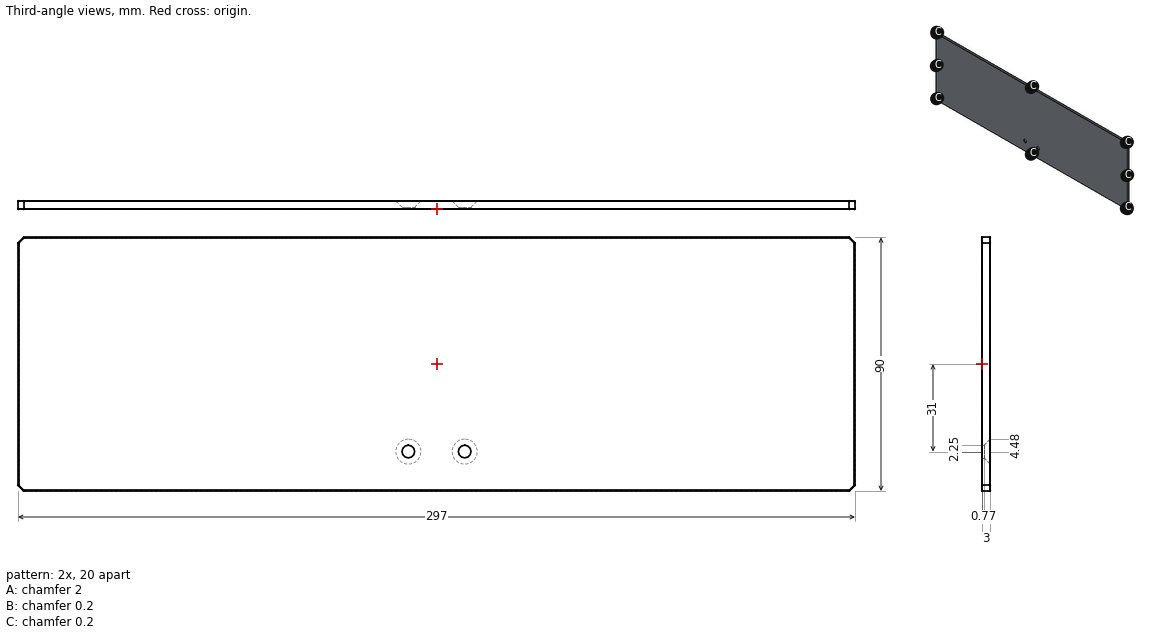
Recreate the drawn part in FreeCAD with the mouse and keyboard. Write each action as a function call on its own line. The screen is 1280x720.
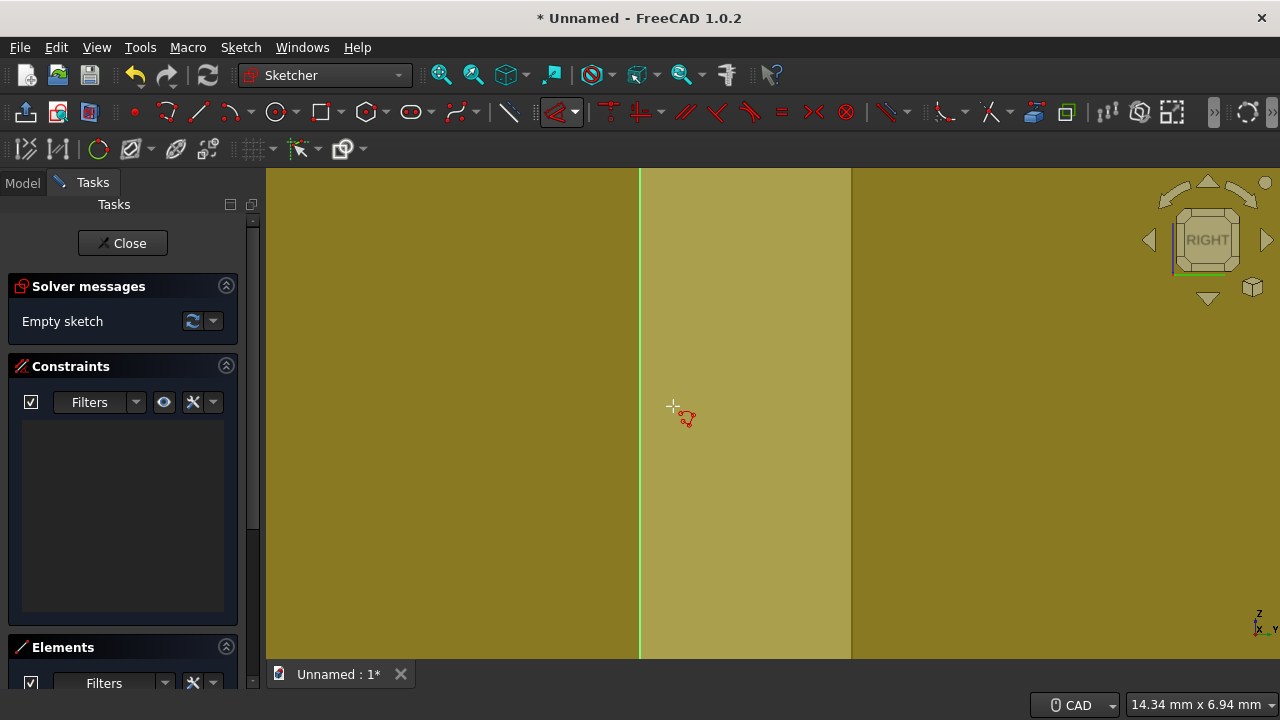
click(852, 255)
click(695, 412)
click(640, 412)
click(649, 571)
click(852, 571)
click(852, 256)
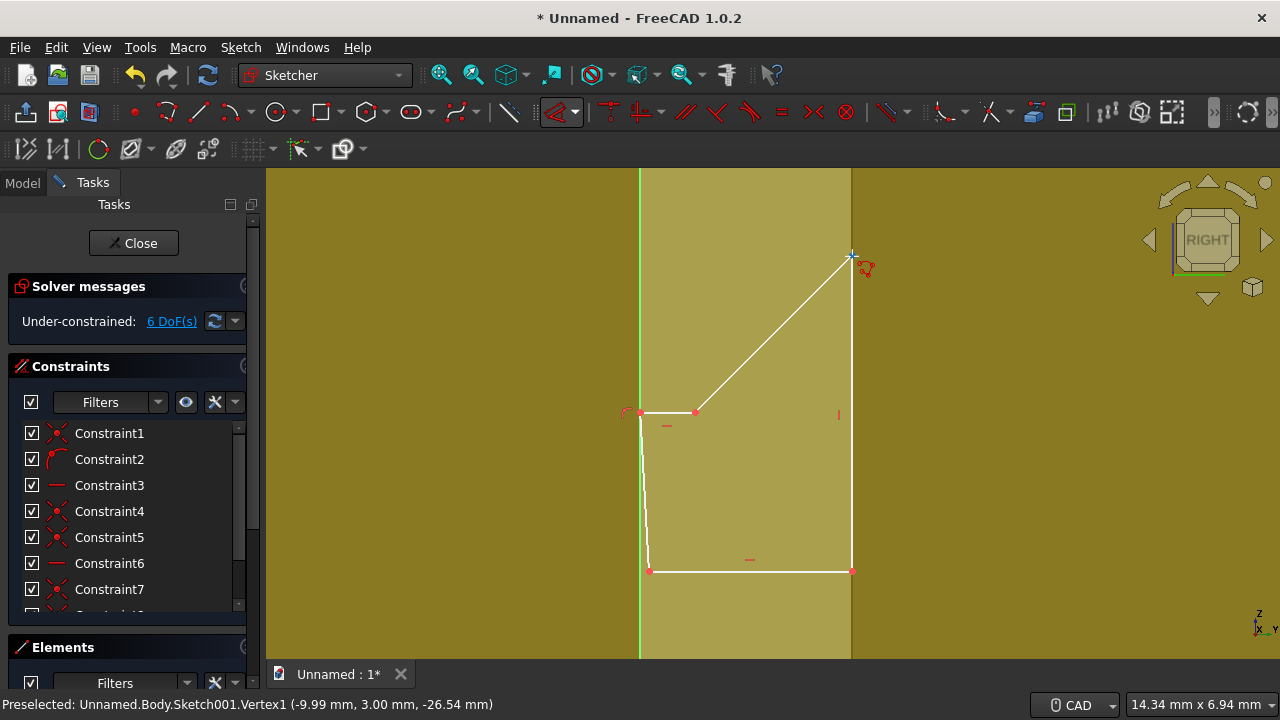
key(g)
key(l)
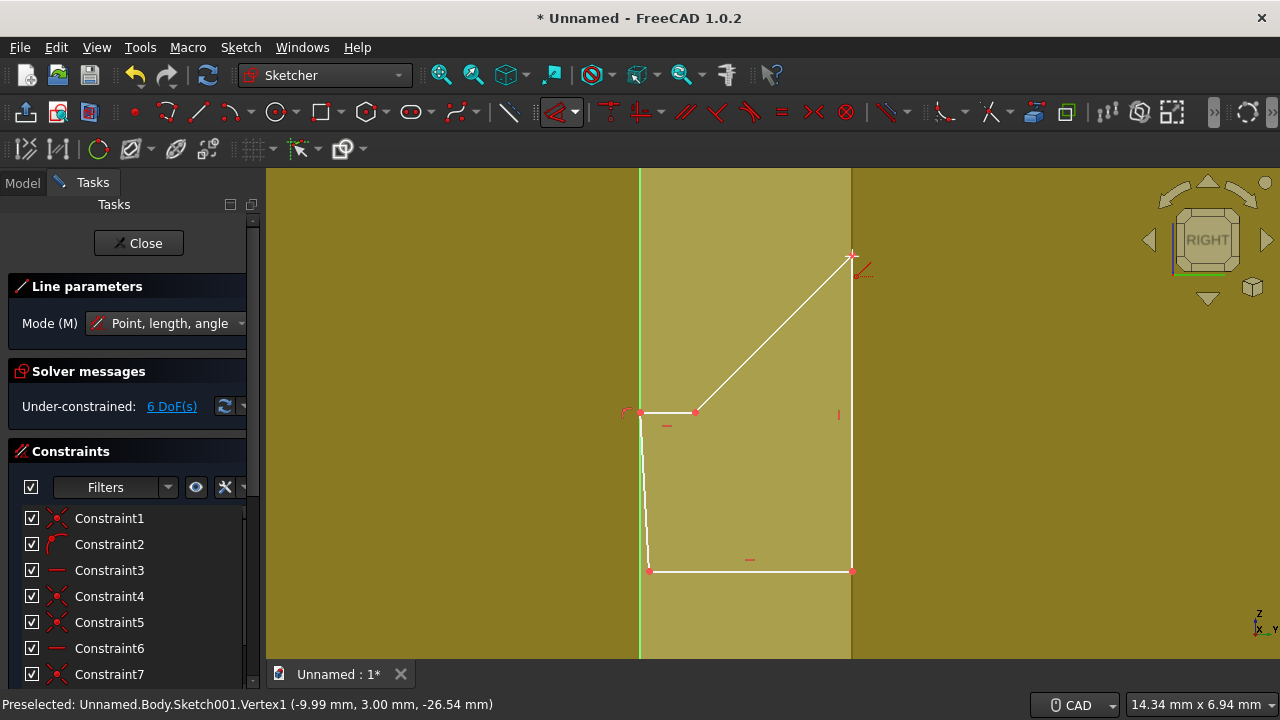
click(619, 571)
click(555, 571)
key(Escape)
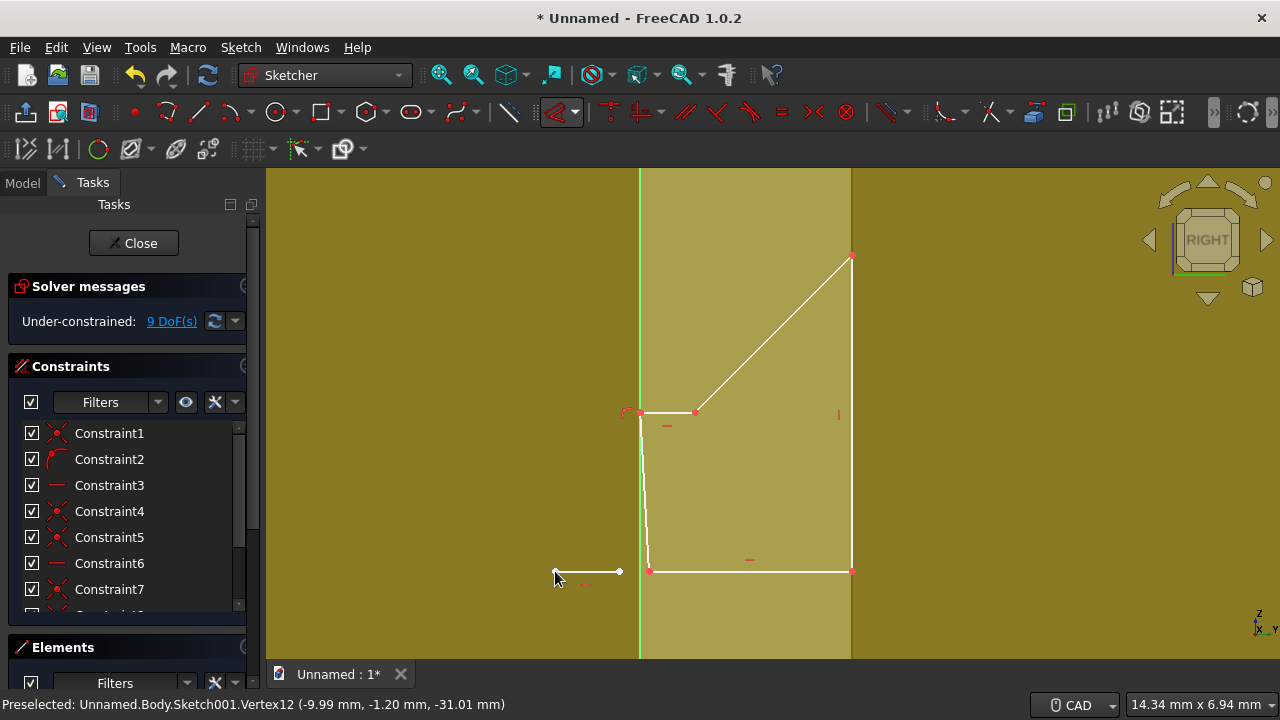
click(600, 572)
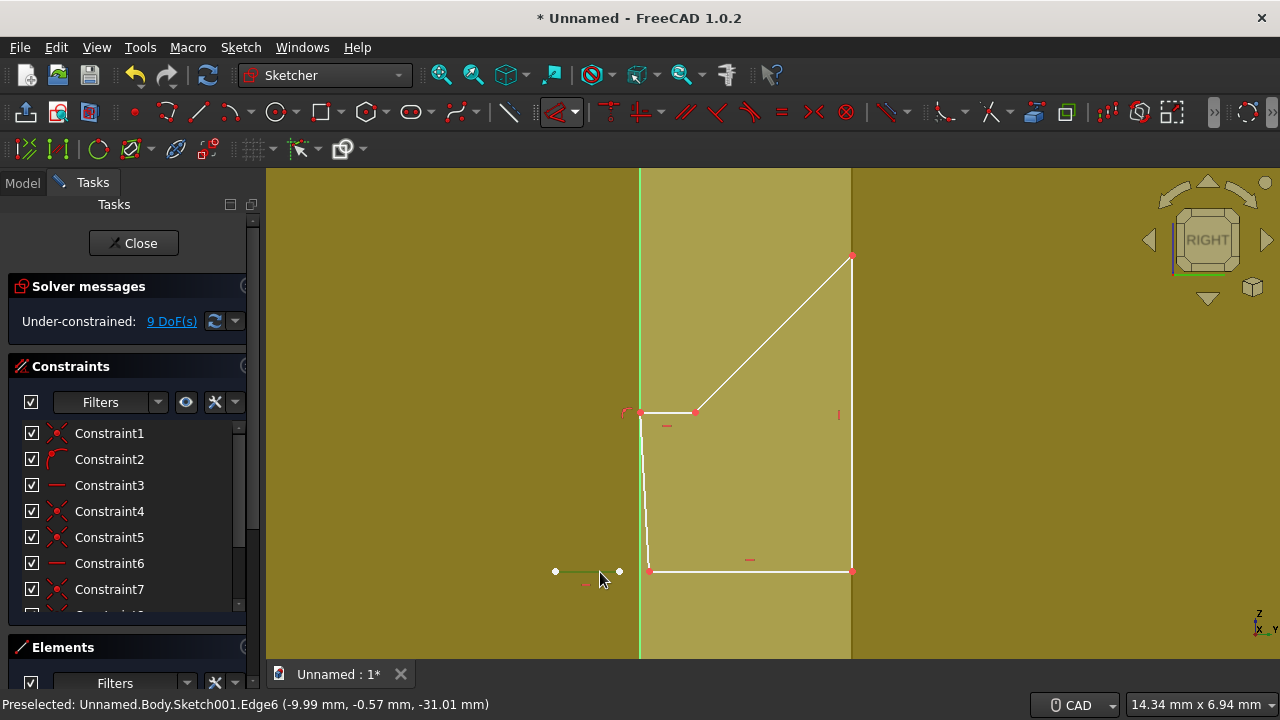
click(510, 112)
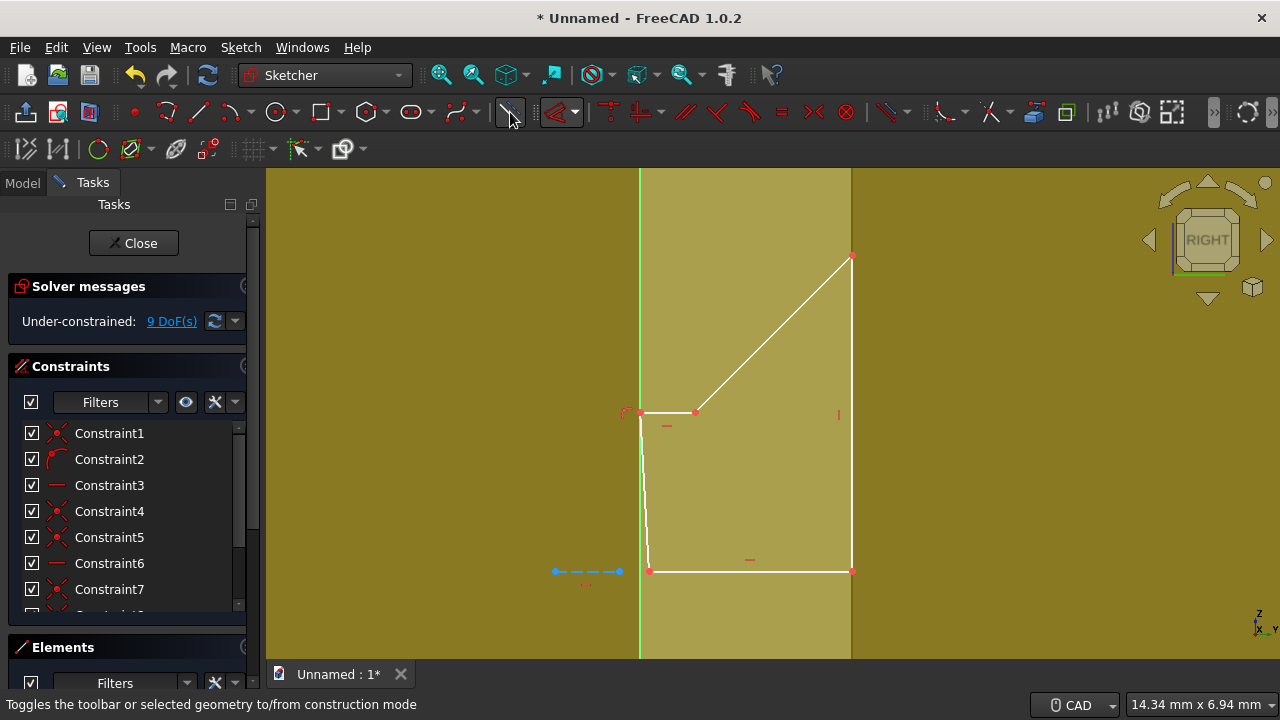
click(643, 461)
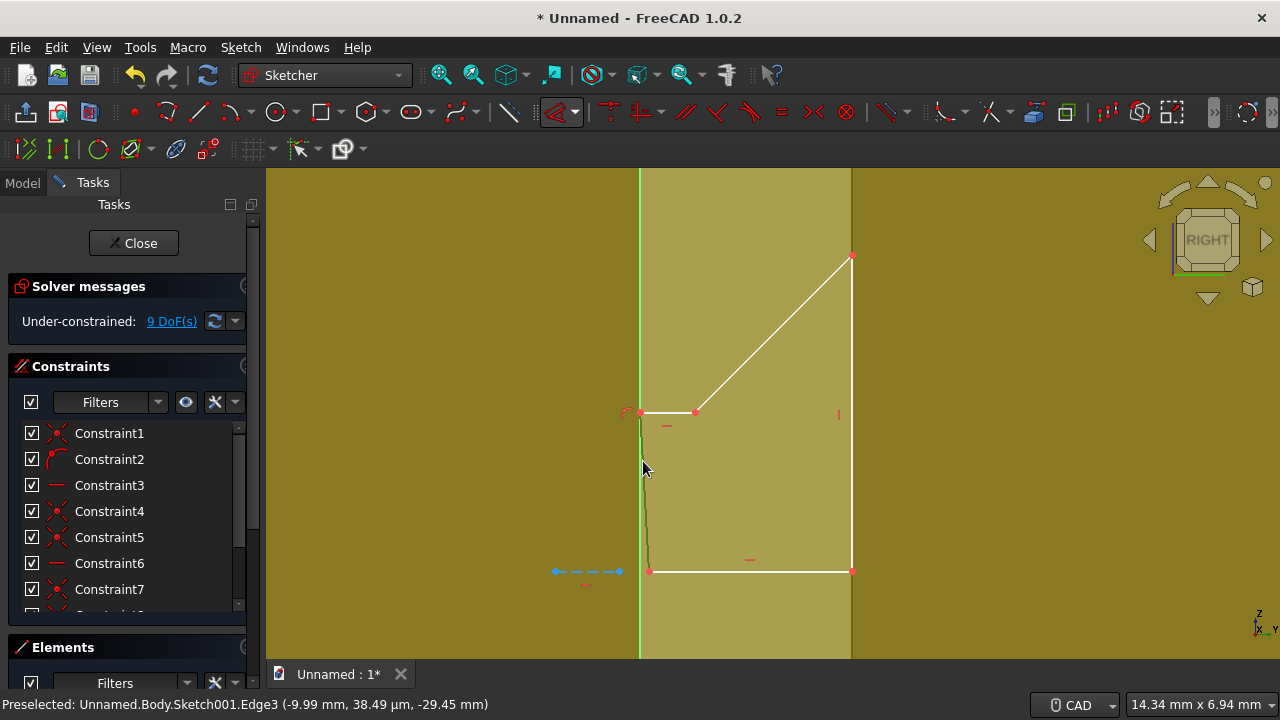
key(v)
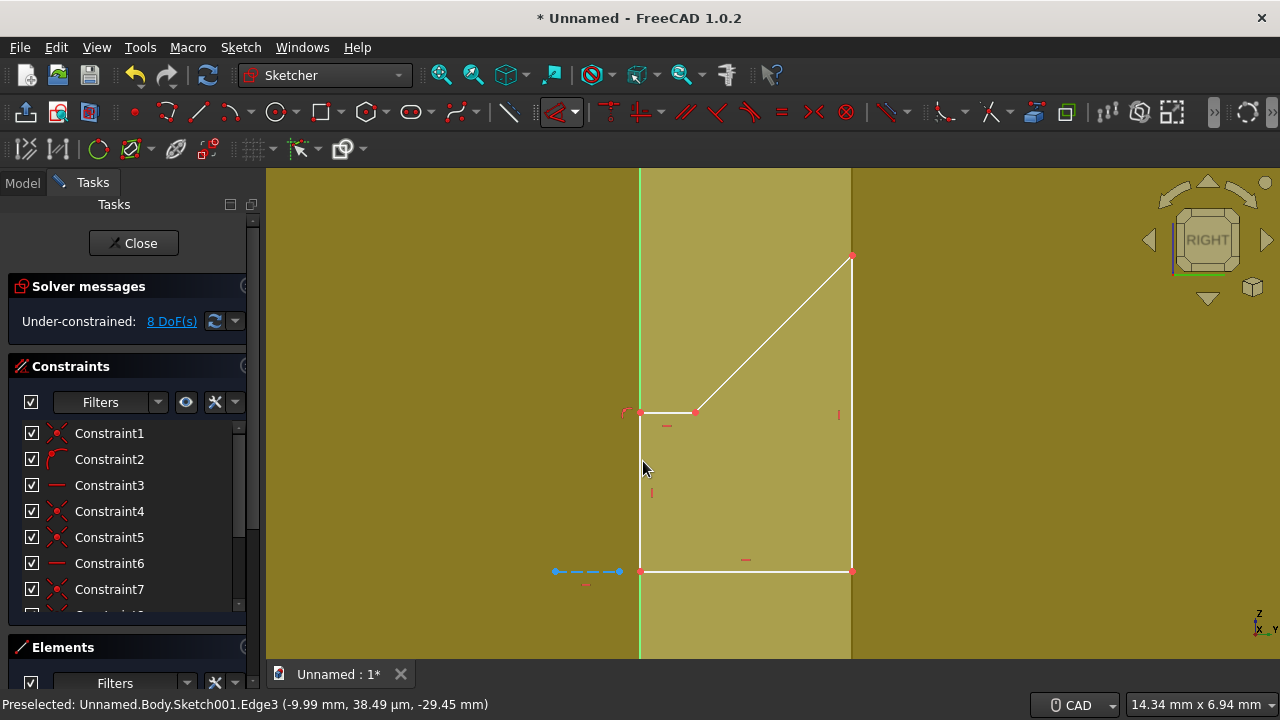
click(704, 572)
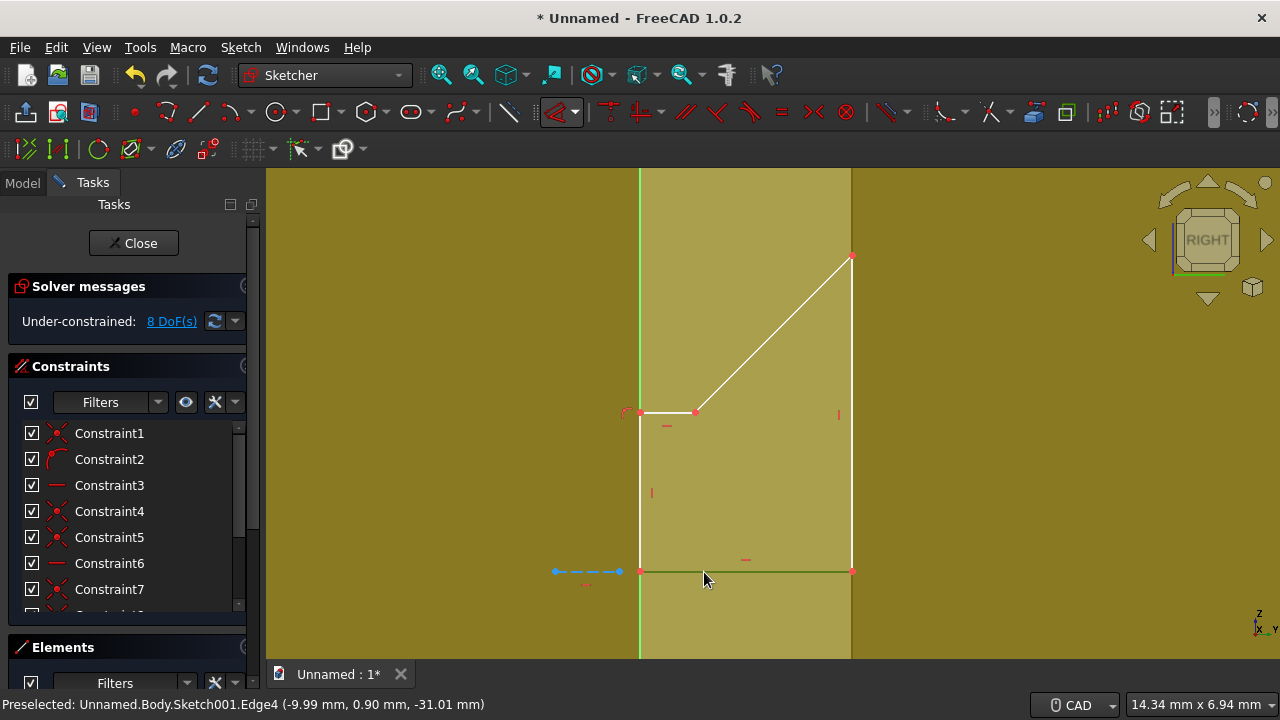
key(l)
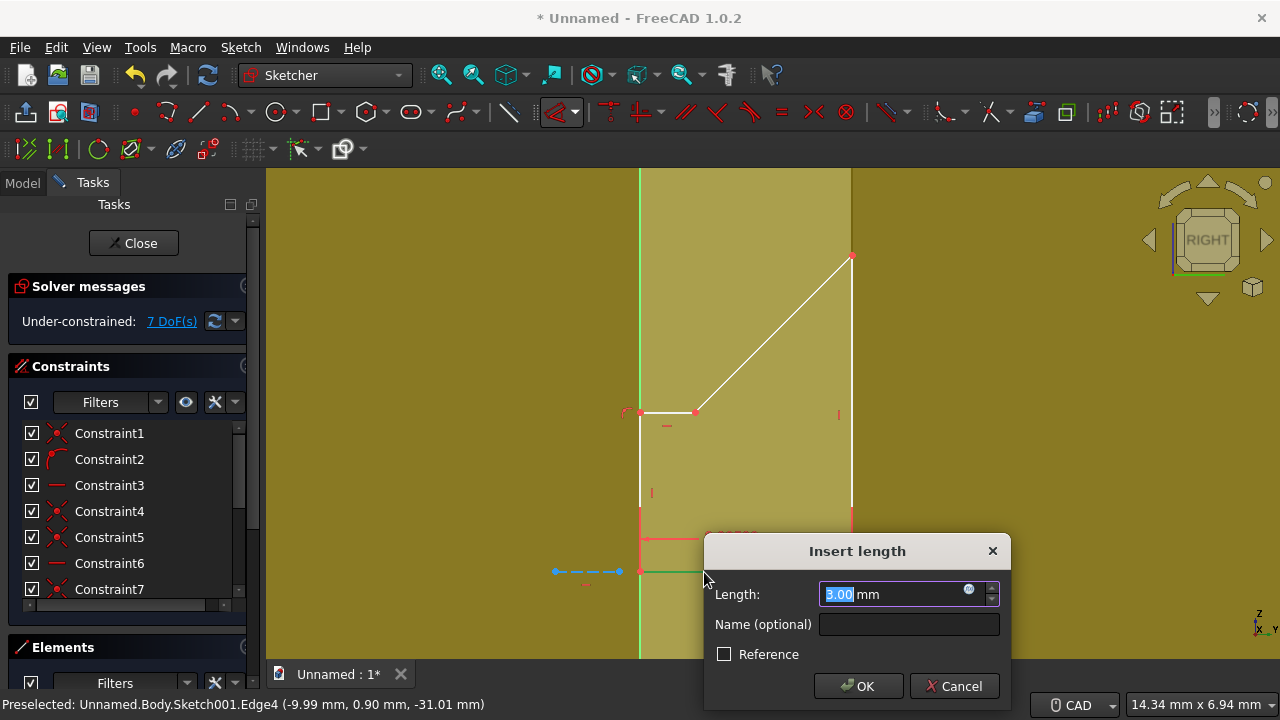
text(3)
key(Return)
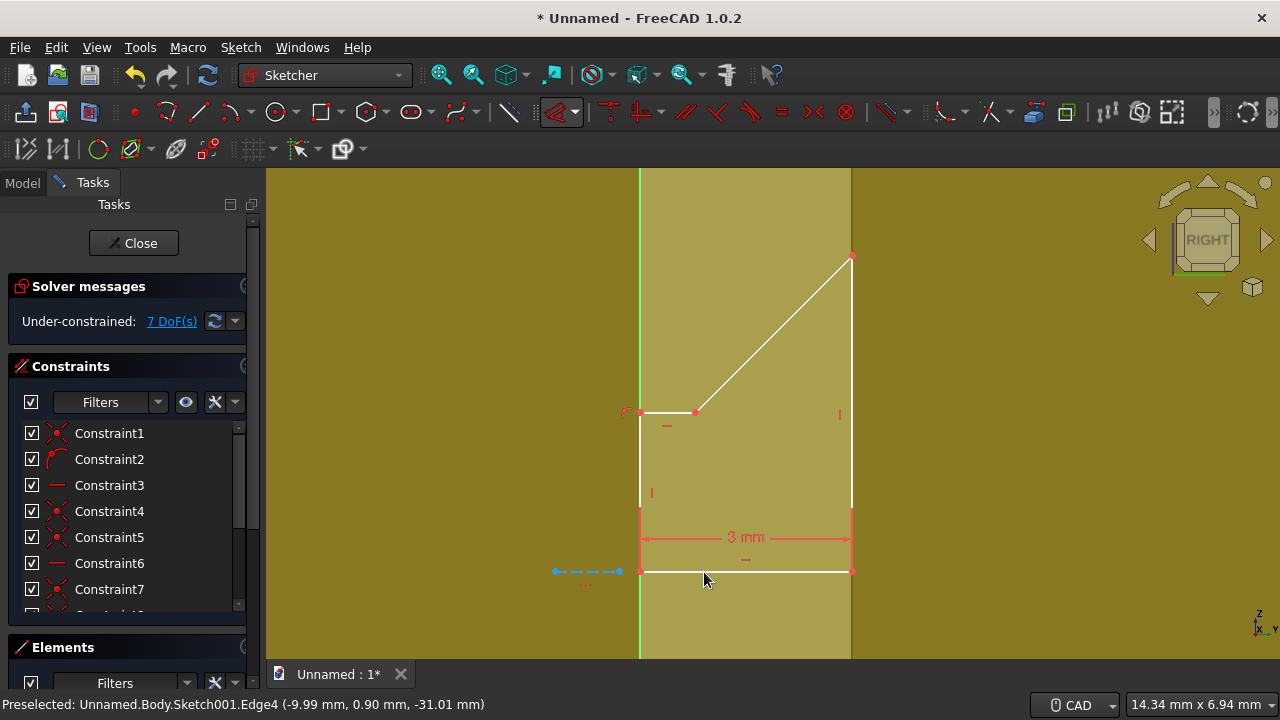
click(640, 572)